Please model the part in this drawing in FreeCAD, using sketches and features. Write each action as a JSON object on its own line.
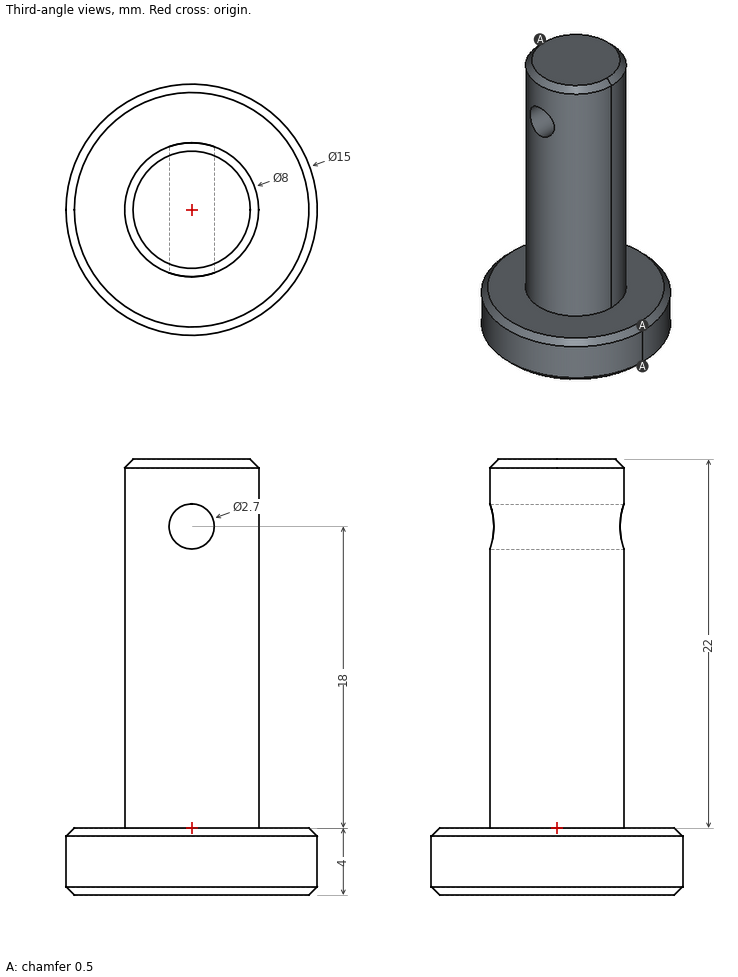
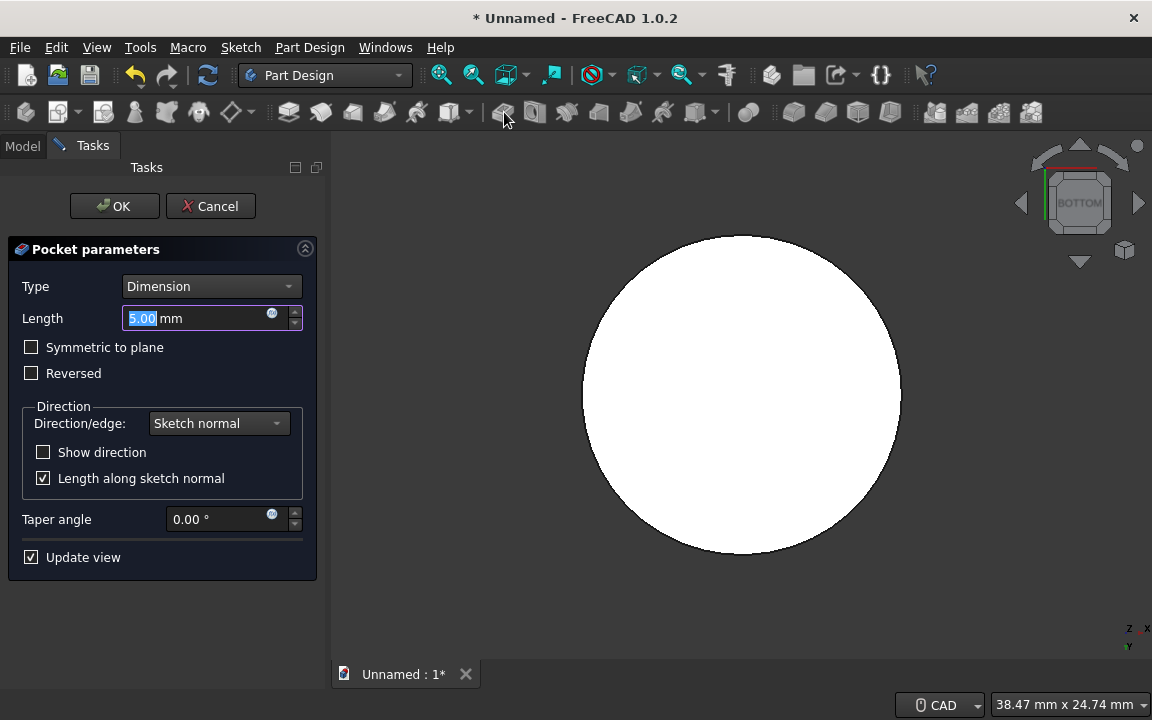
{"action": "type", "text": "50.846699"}
{"action": "key", "text": "Tab"}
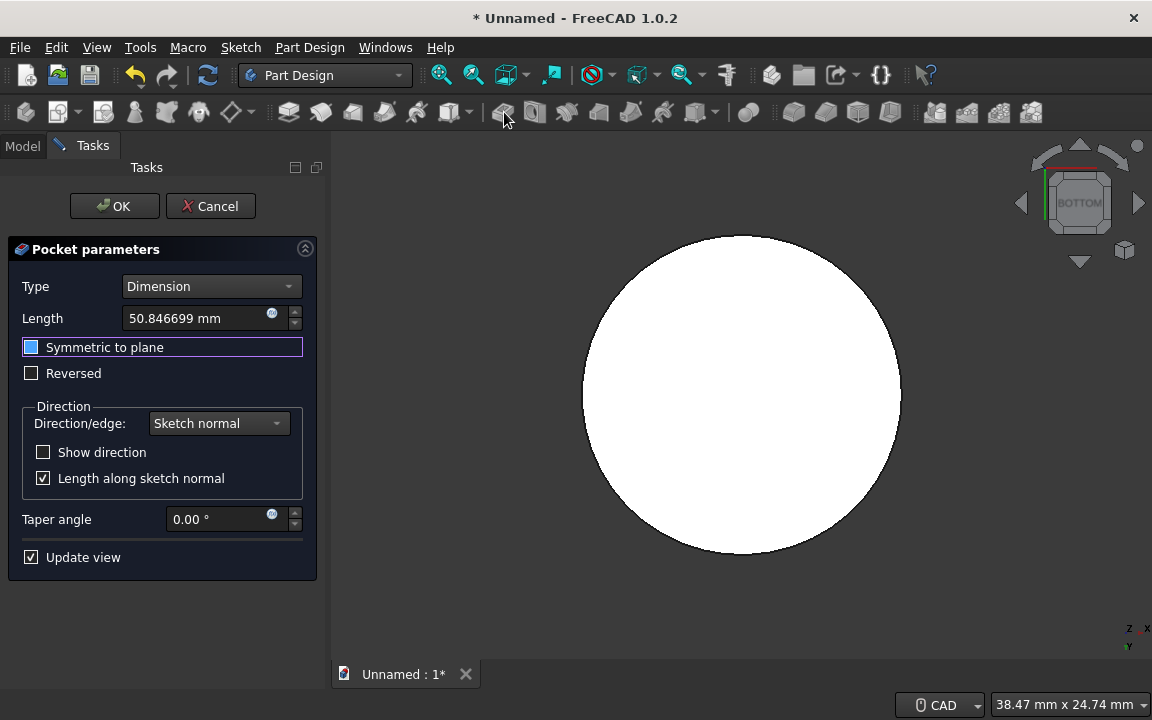
{"action": "left_click", "coordinate": [30, 347]}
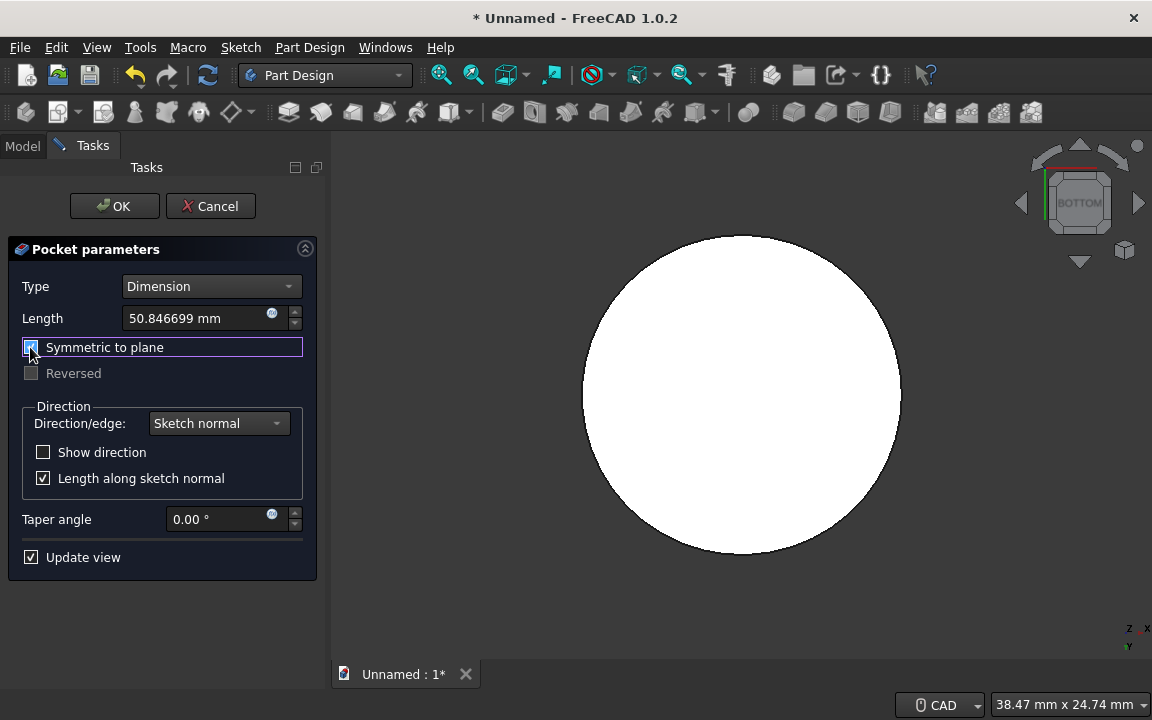
{"action": "left_click", "coordinate": [115, 206]}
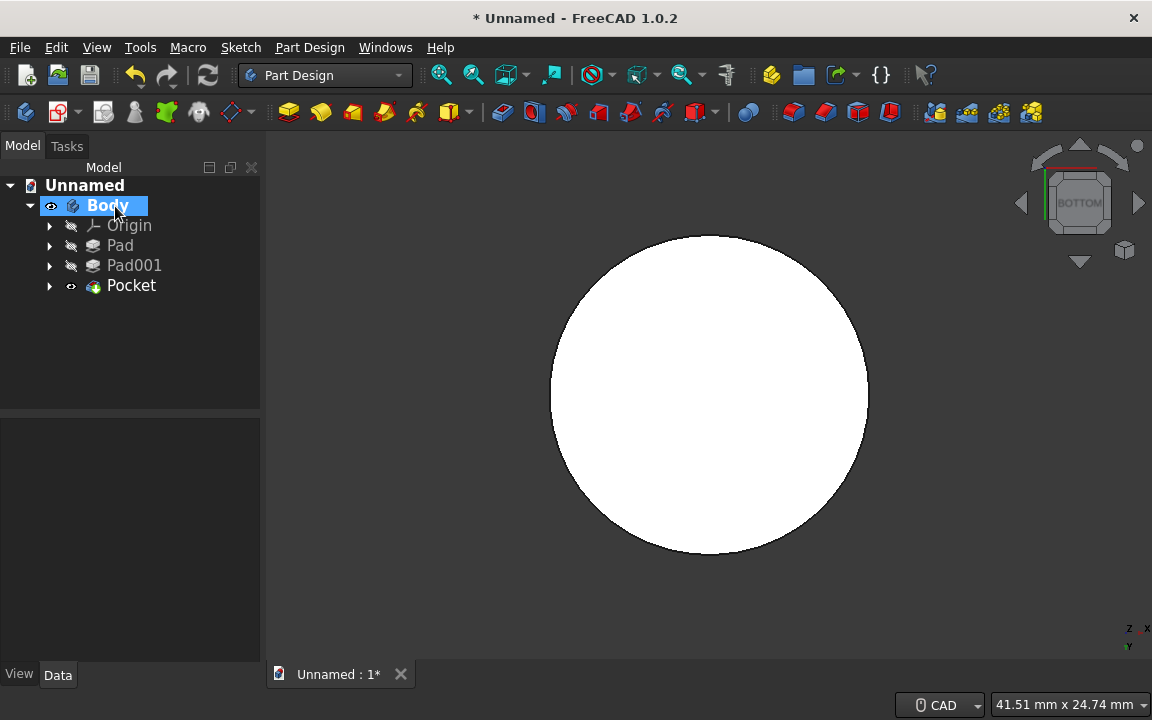
{"action": "left_click", "coordinate": [549, 394]}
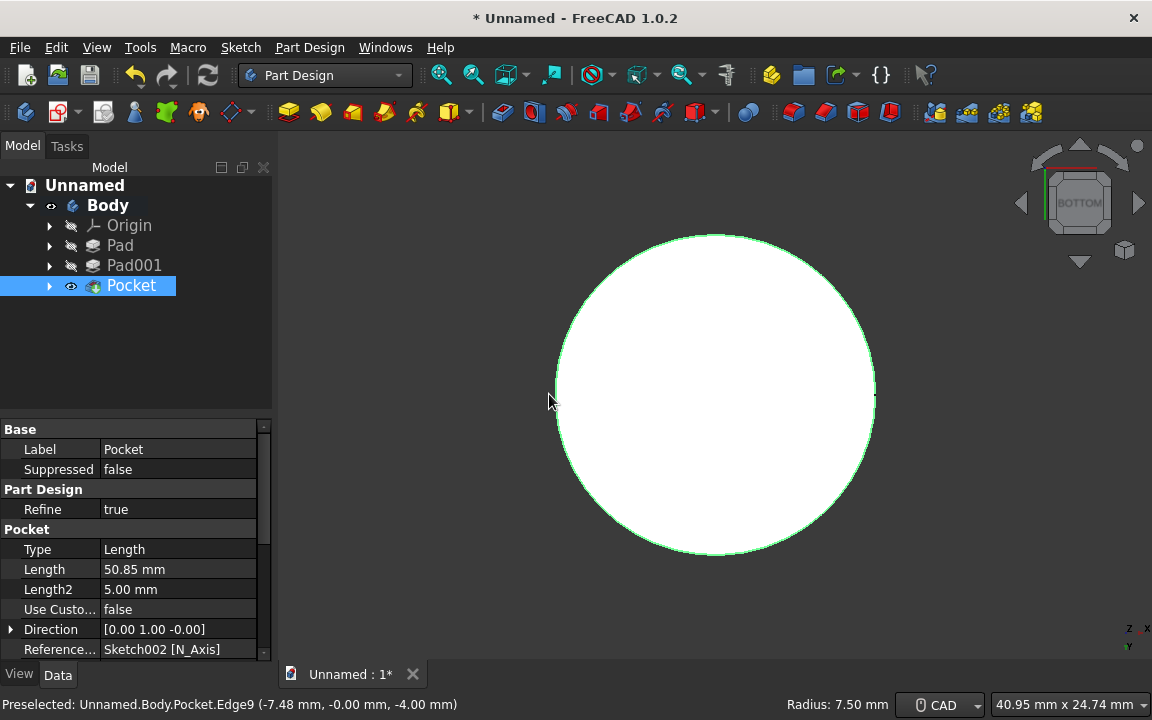
{"action": "key", "text": "0"}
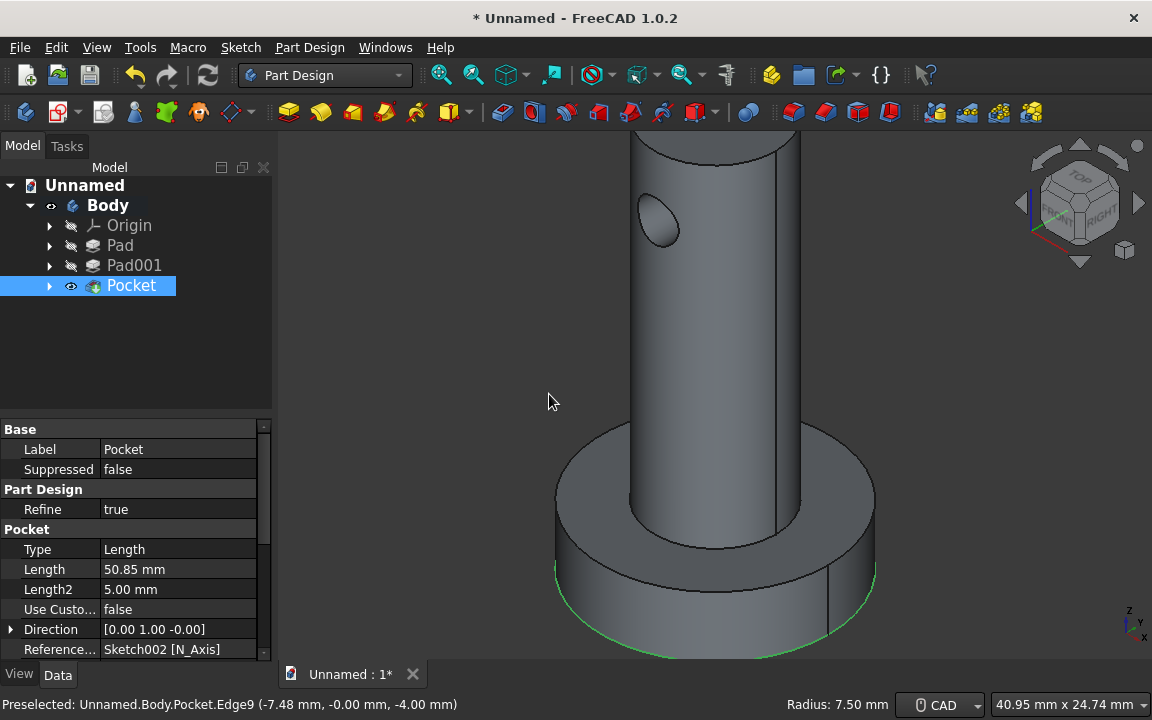
{"action": "left_click", "coordinate": [442, 76]}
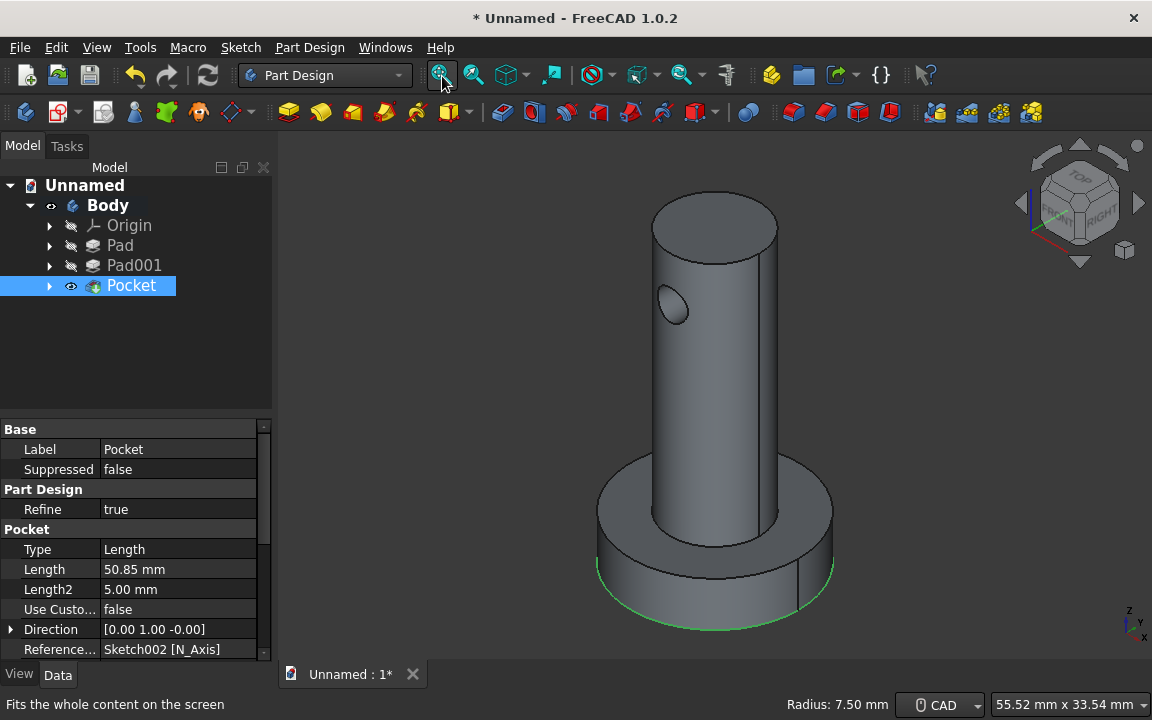
{"action": "left_click", "coordinate": [653, 221], "text": "ctrl"}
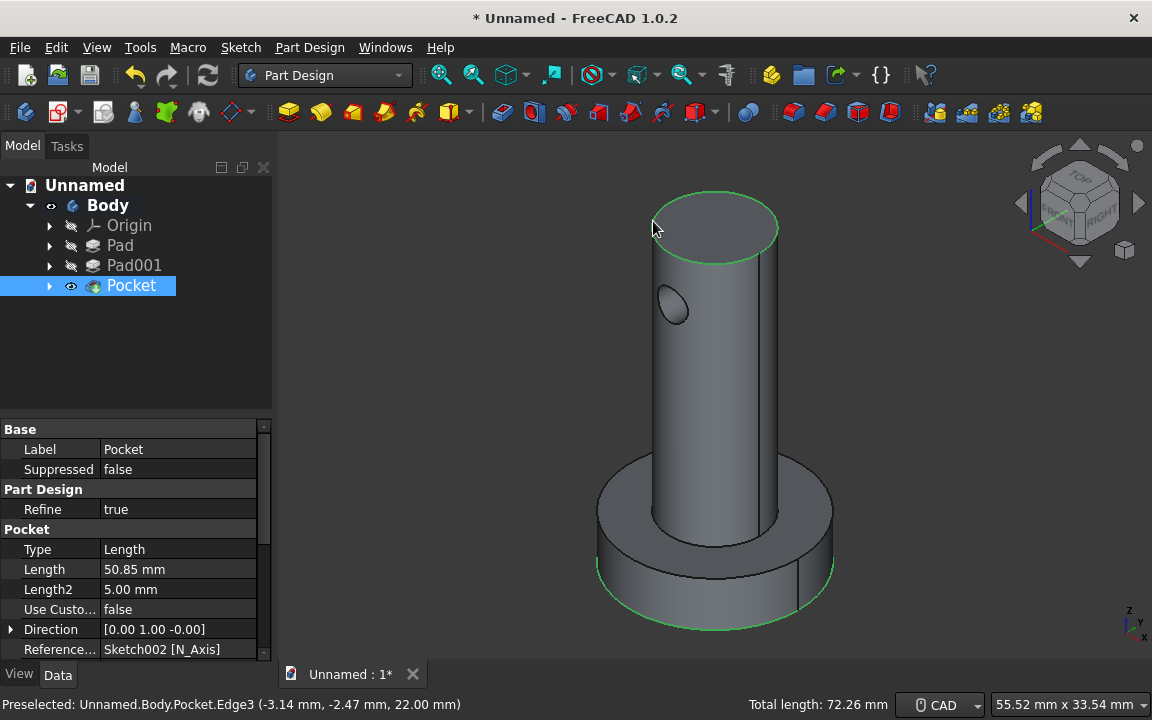
{"action": "left_click", "coordinate": [610, 541], "text": "ctrl"}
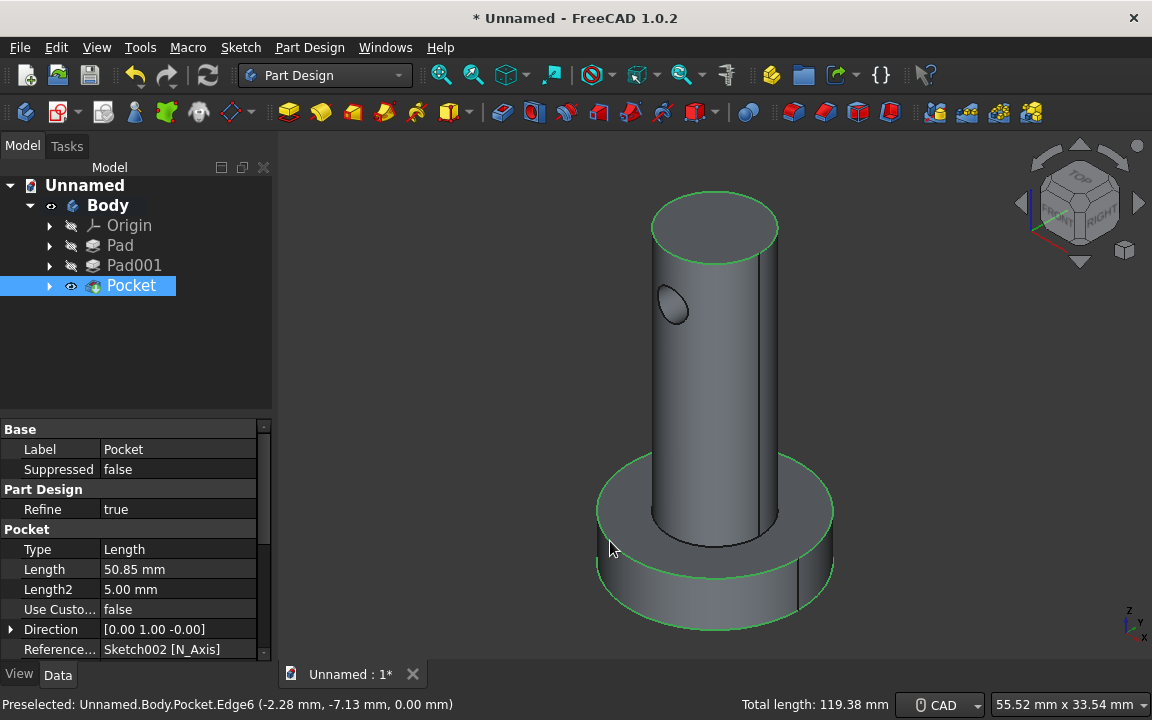
{"action": "left_click", "coordinate": [826, 112]}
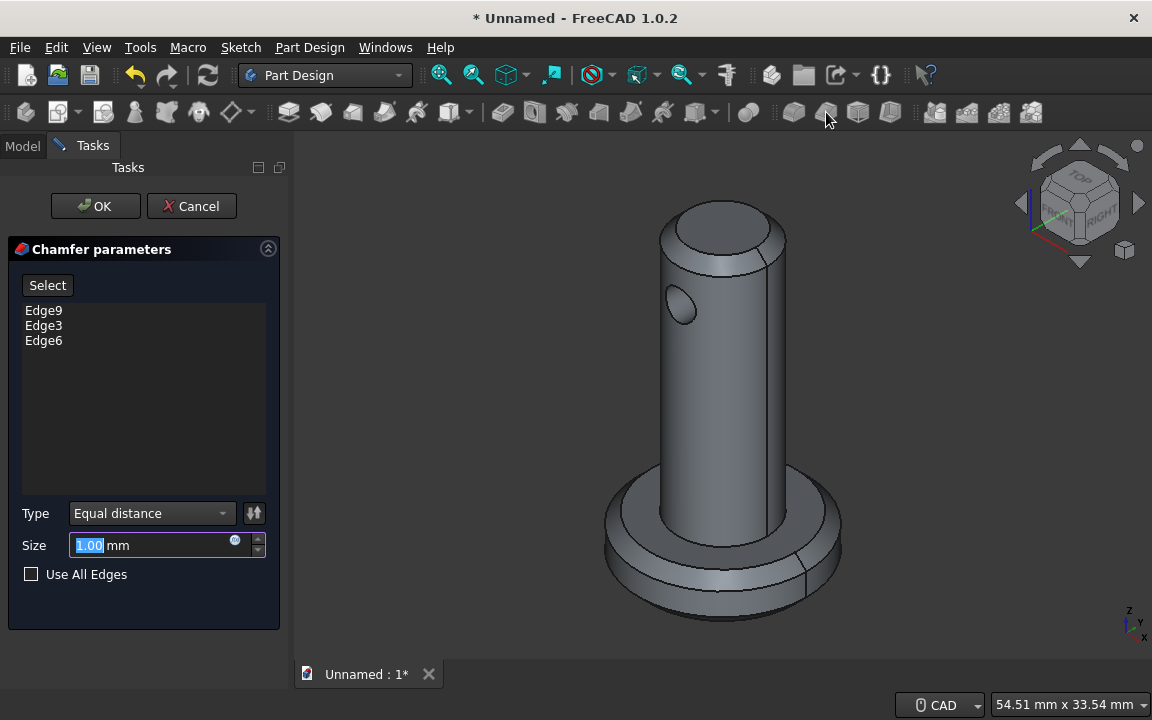
{"action": "type", "text": "0.5"}
{"action": "key", "text": "Tab"}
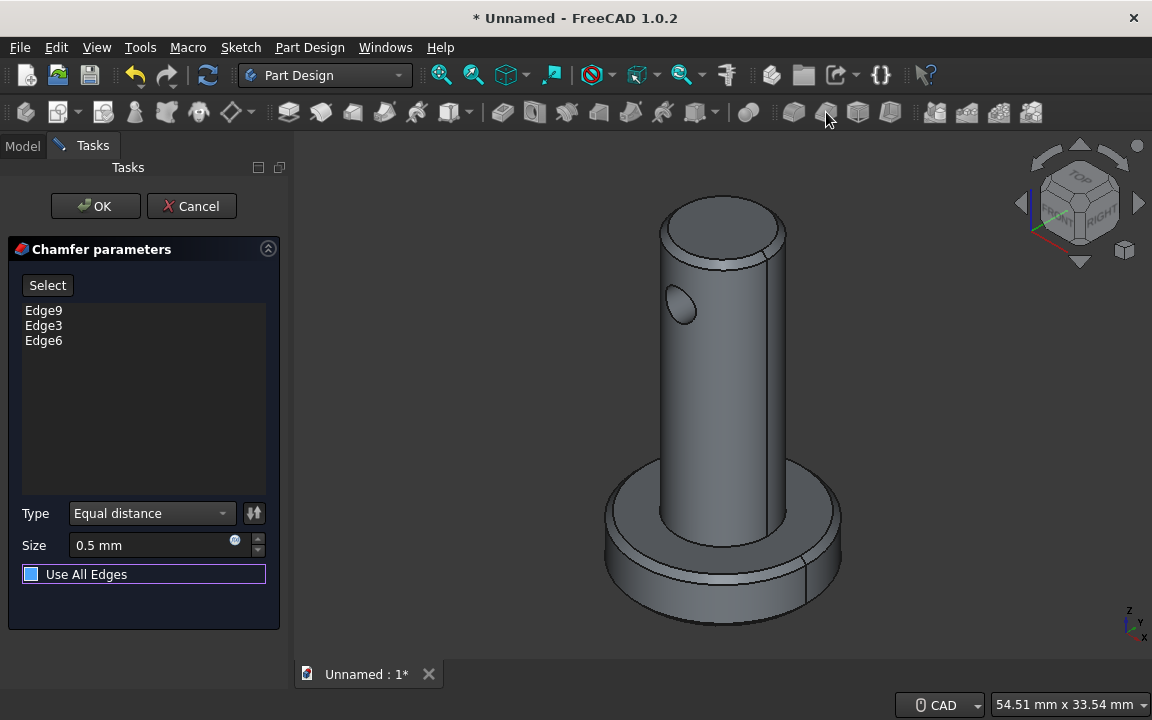
{"action": "left_click", "coordinate": [96, 206]}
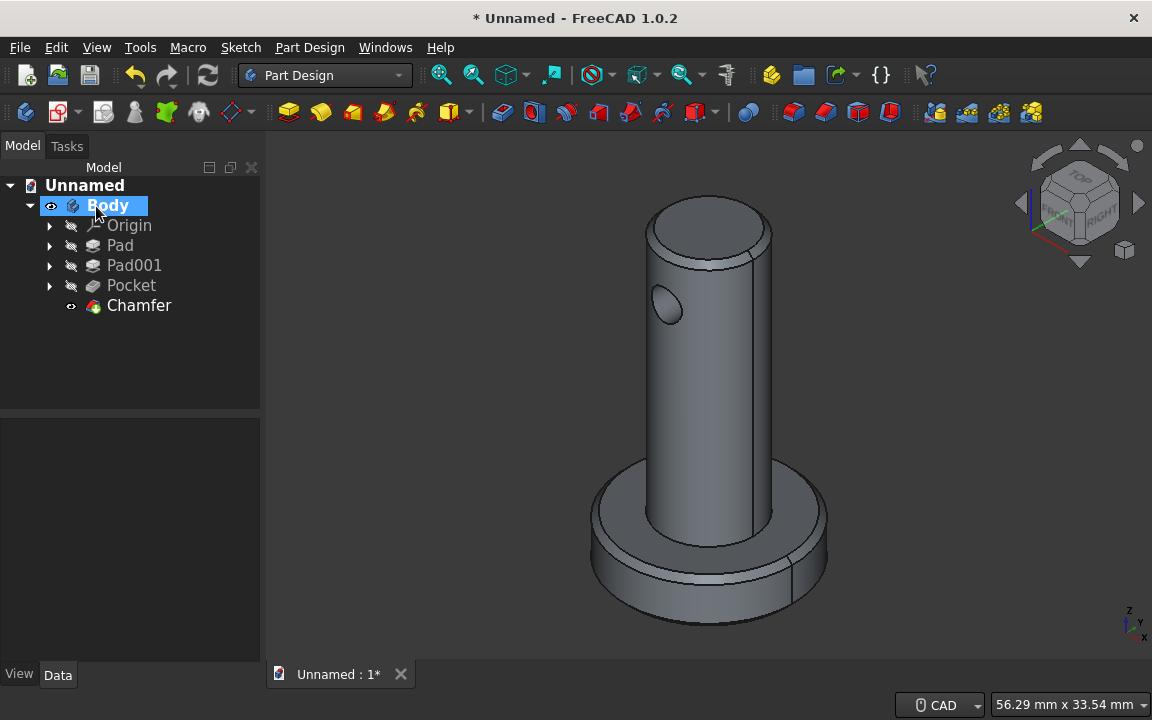
{"action": "left_click", "coordinate": [442, 76]}